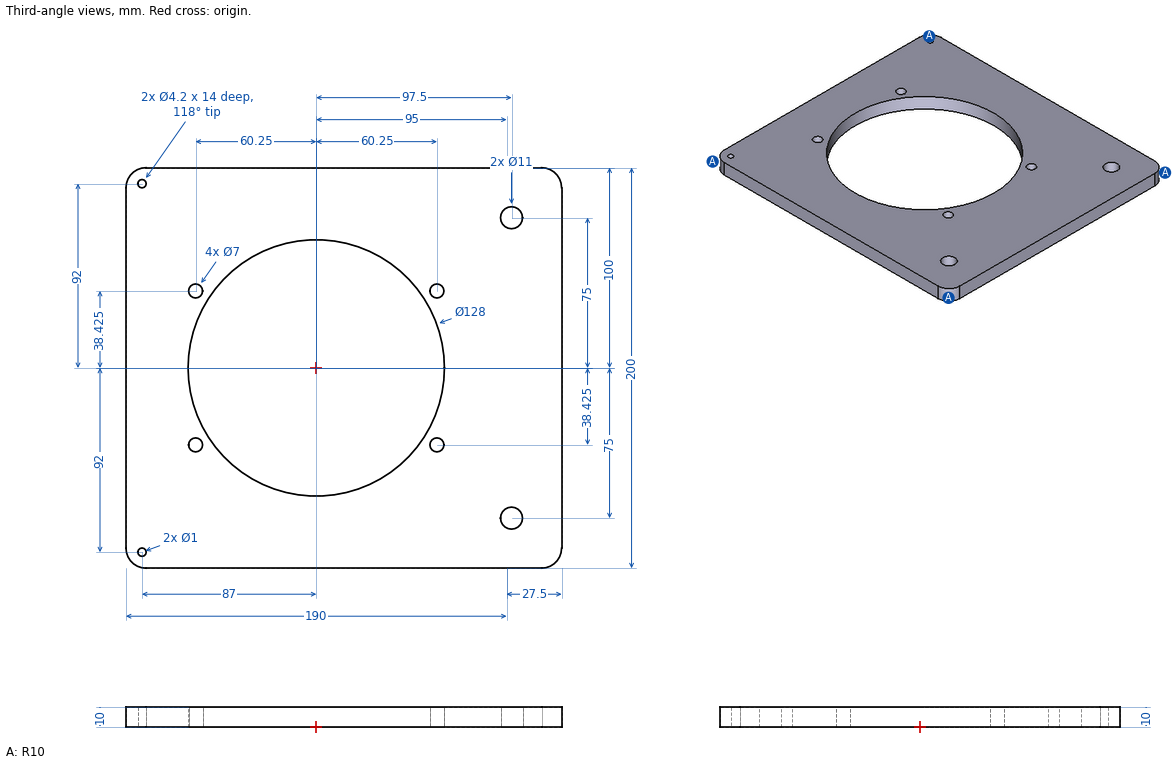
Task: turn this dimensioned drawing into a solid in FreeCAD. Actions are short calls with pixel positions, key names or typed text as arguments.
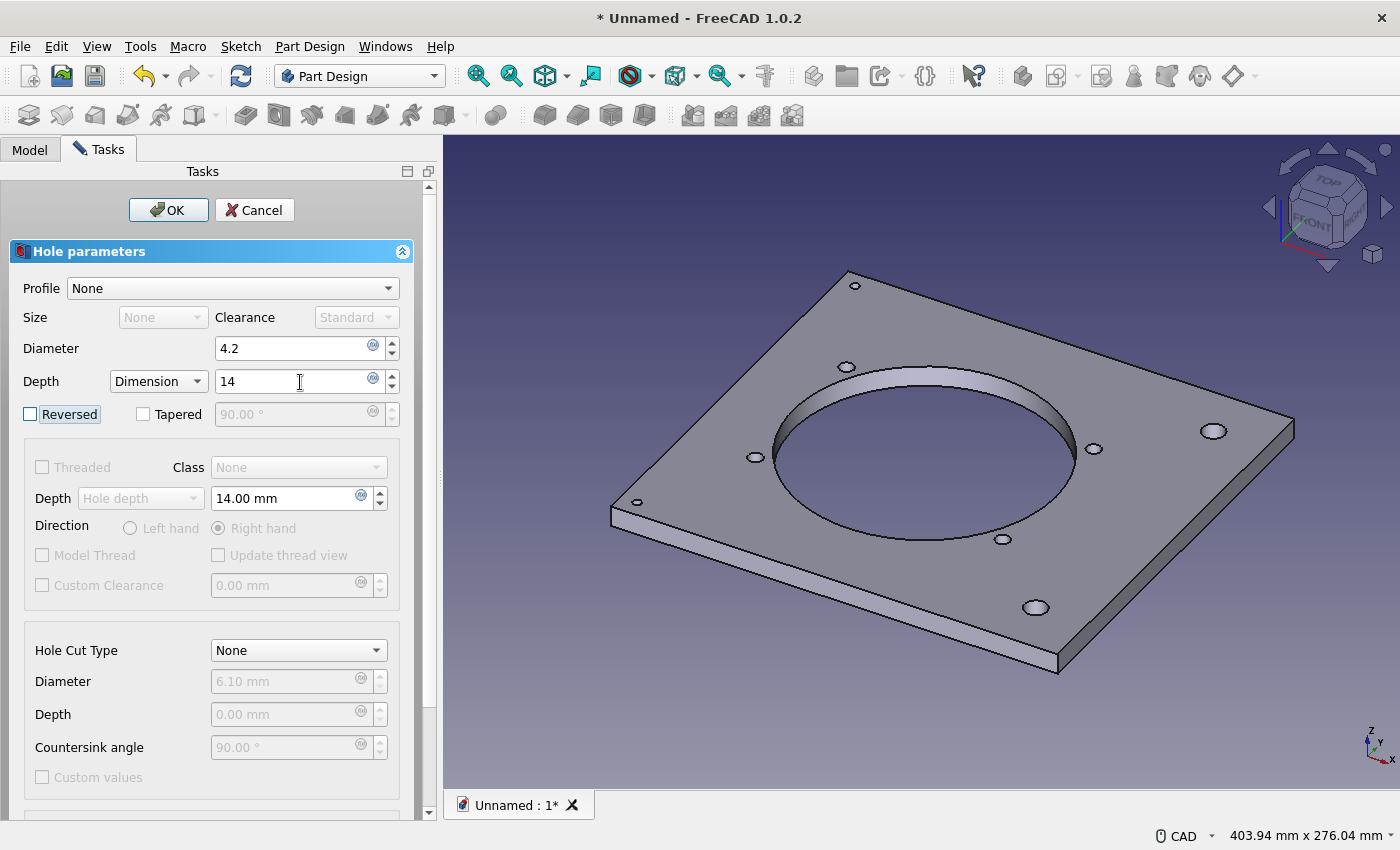
click(169, 210)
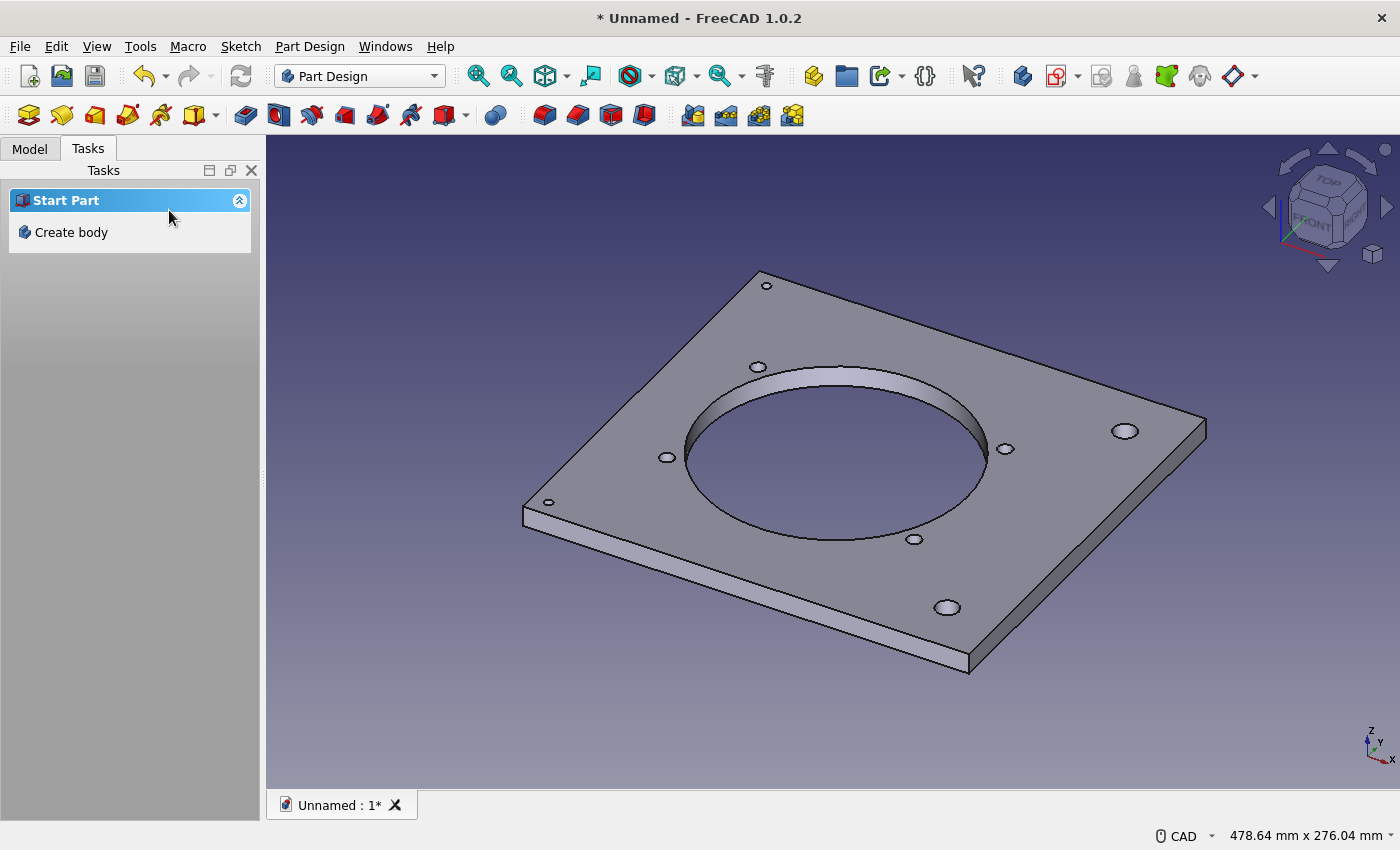
click(969, 663)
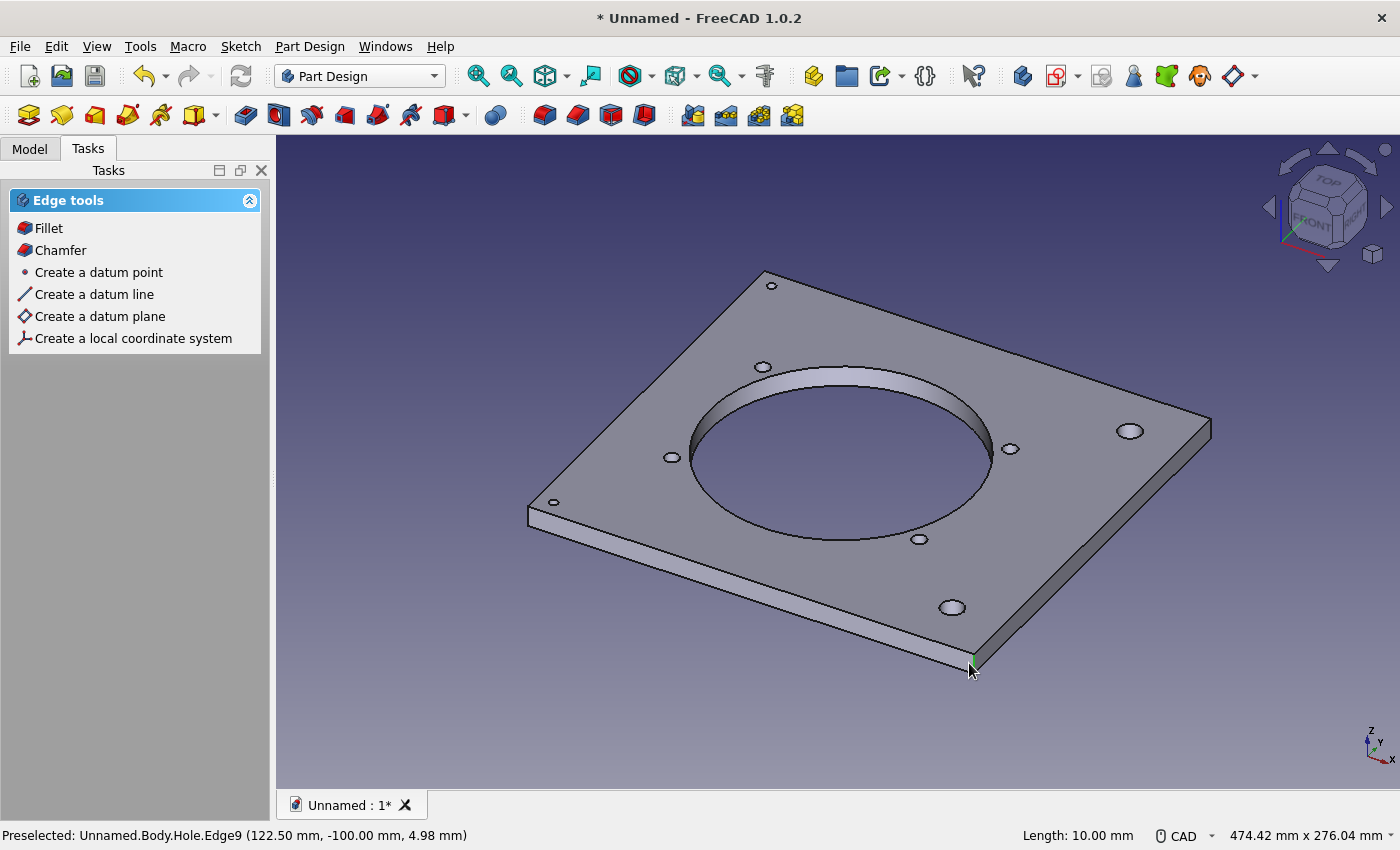
key(0)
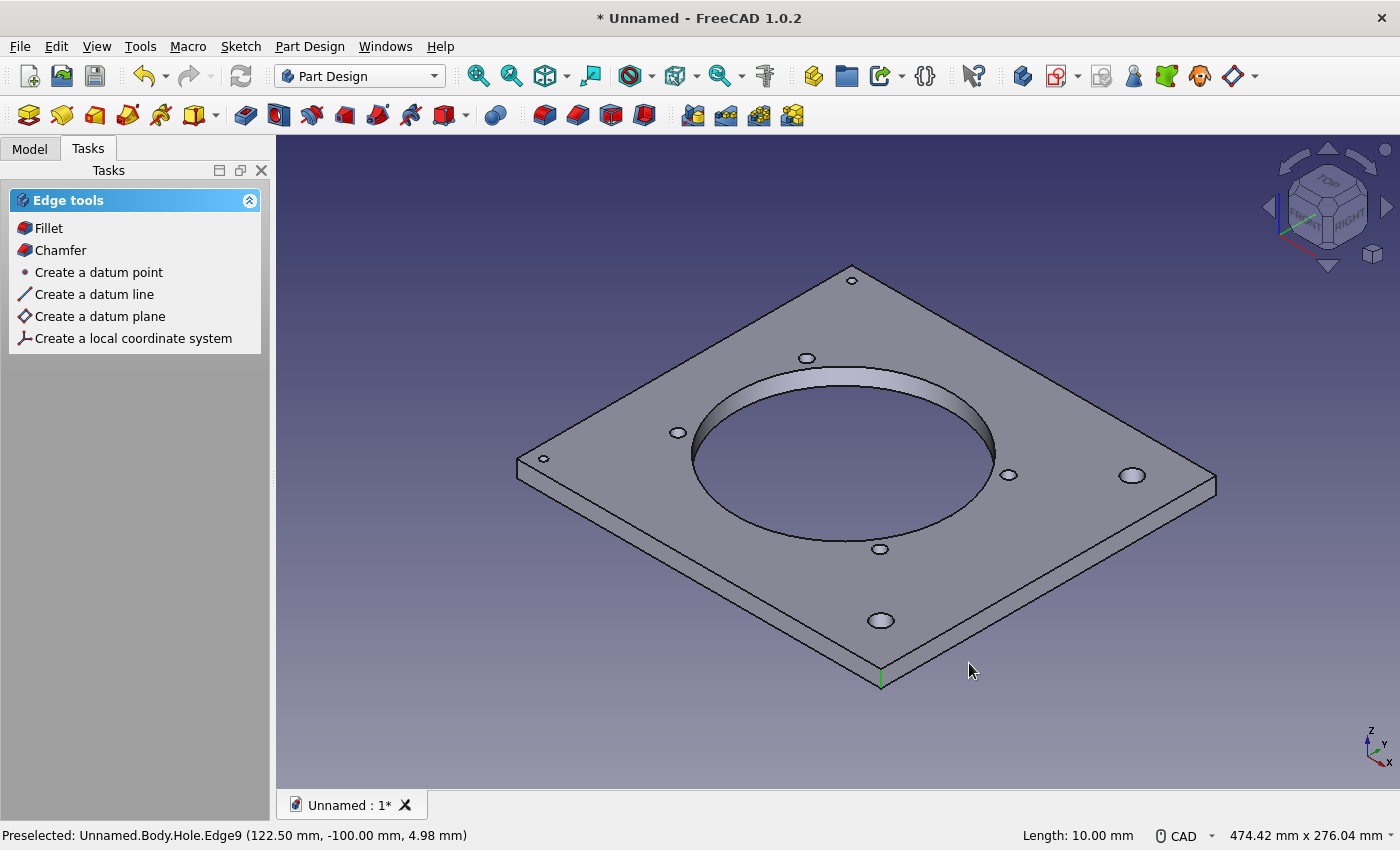
key(2)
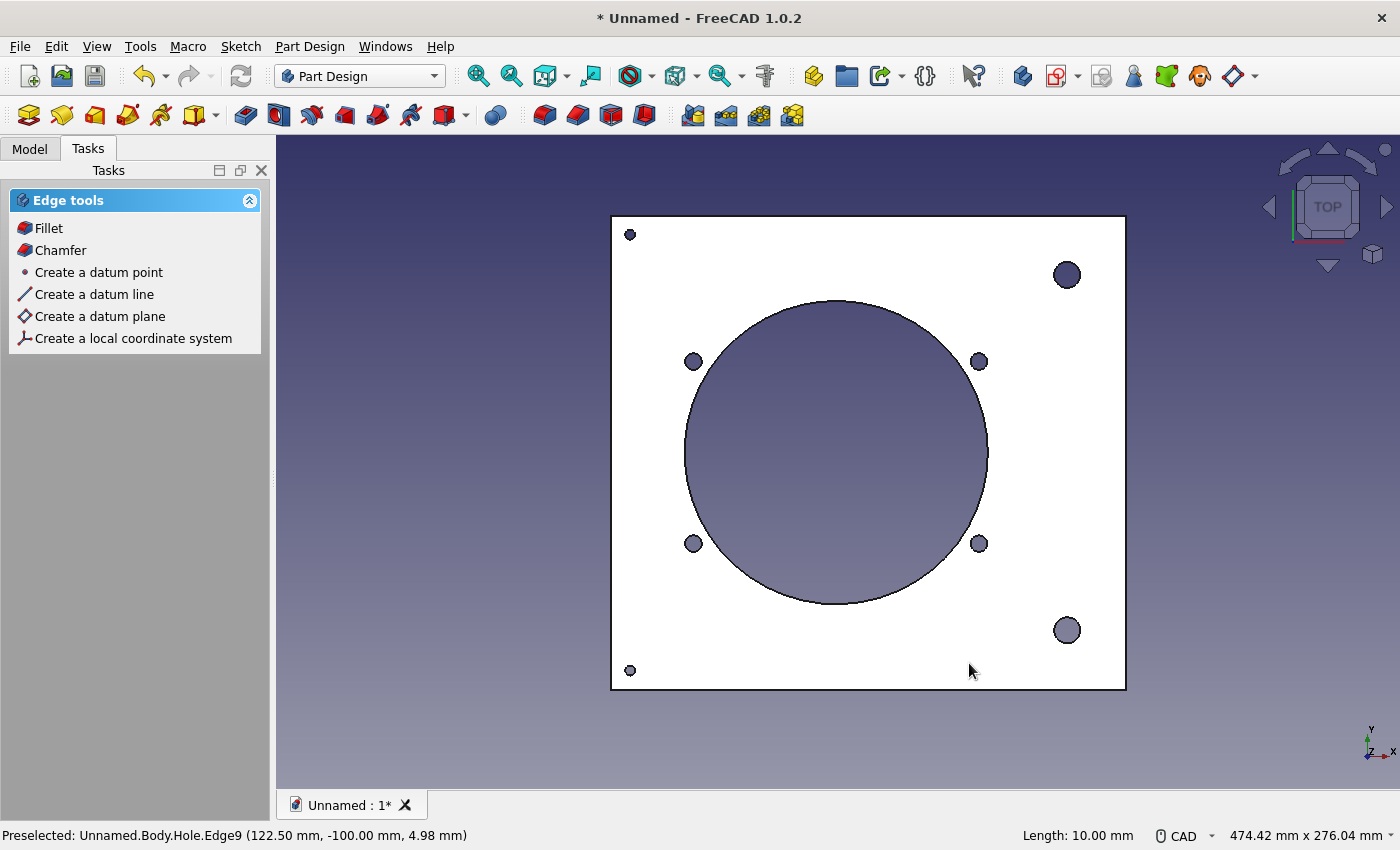
key(1)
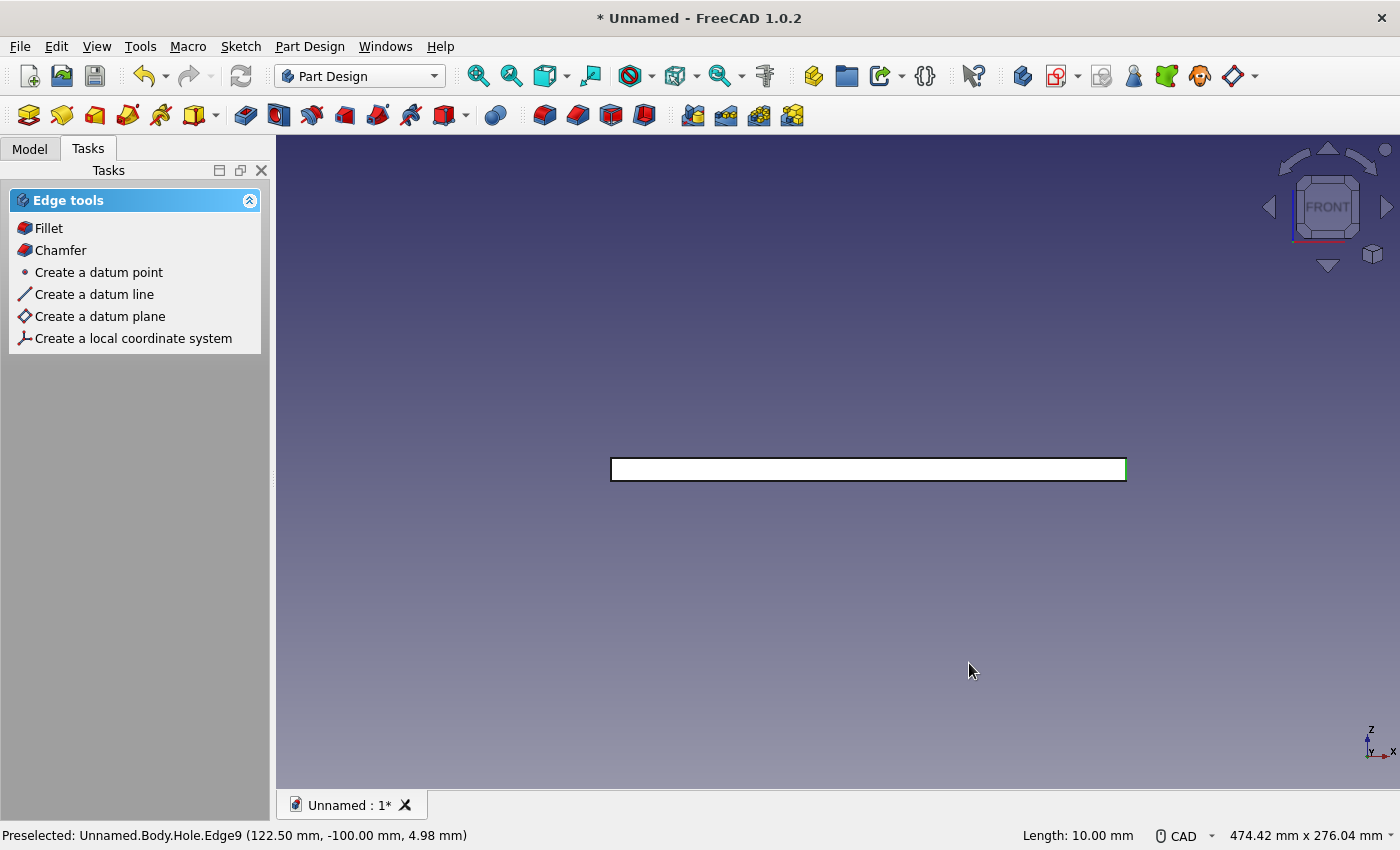
click(611, 469, ctrl)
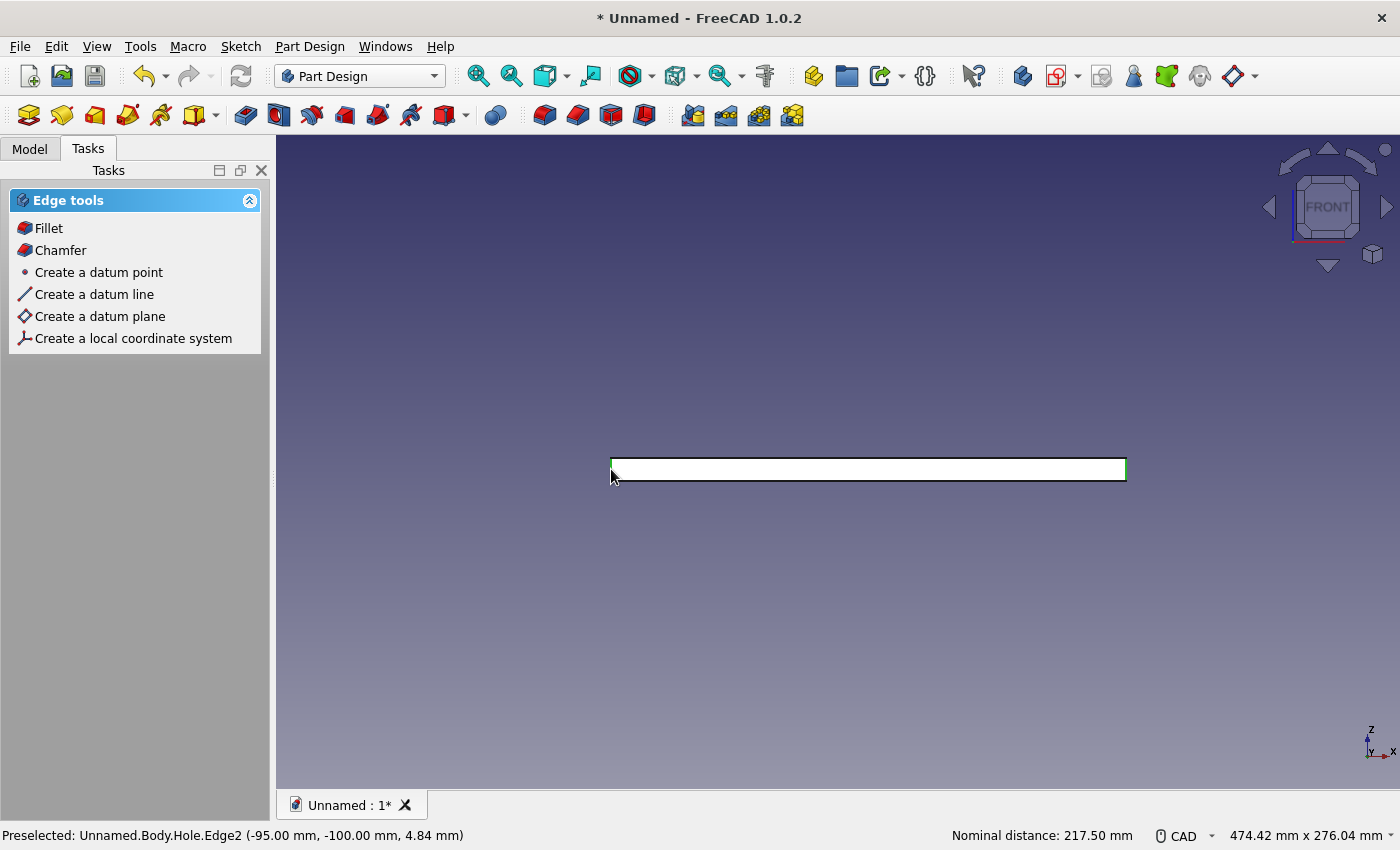
key(3)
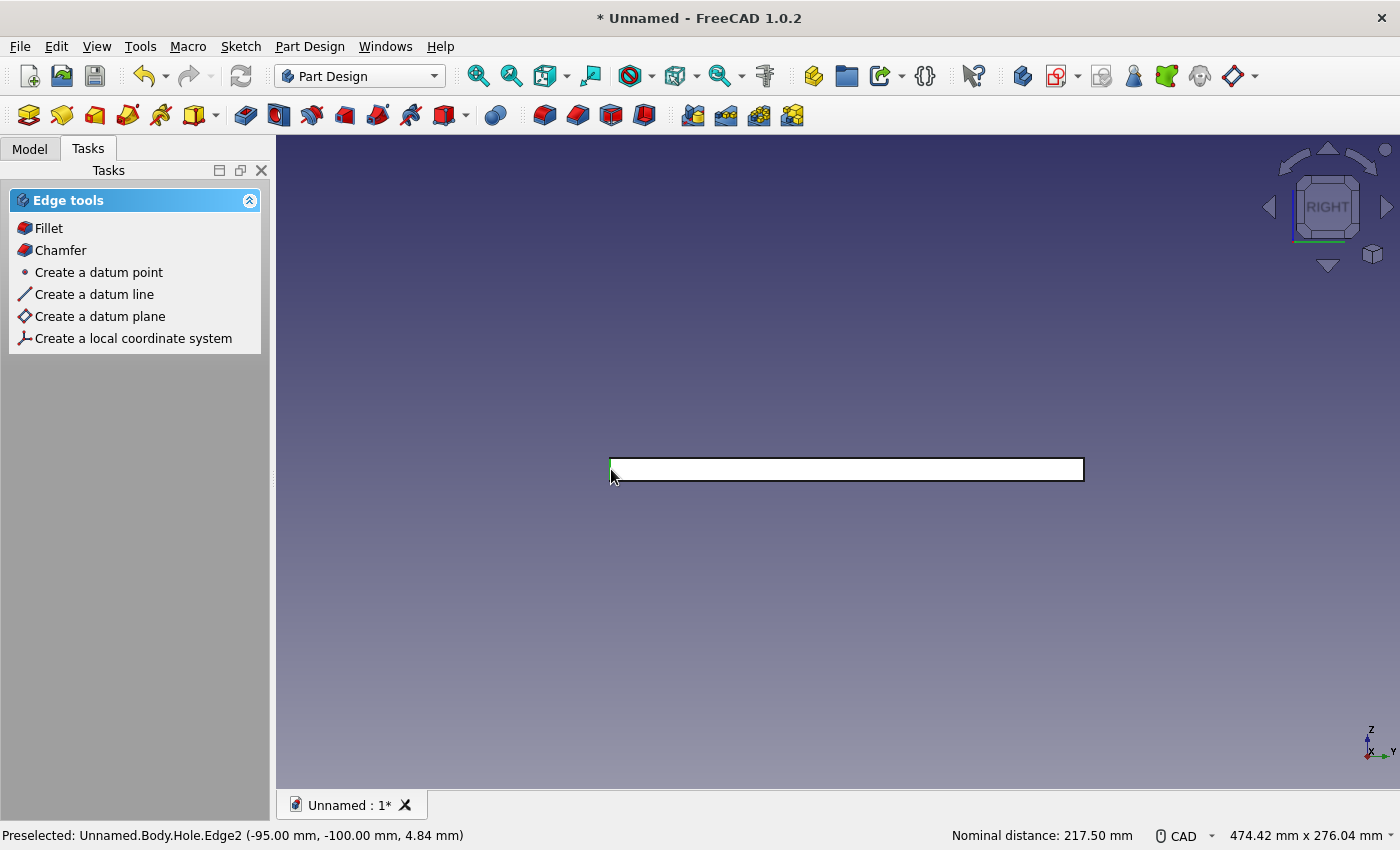
key(v)
key(f)